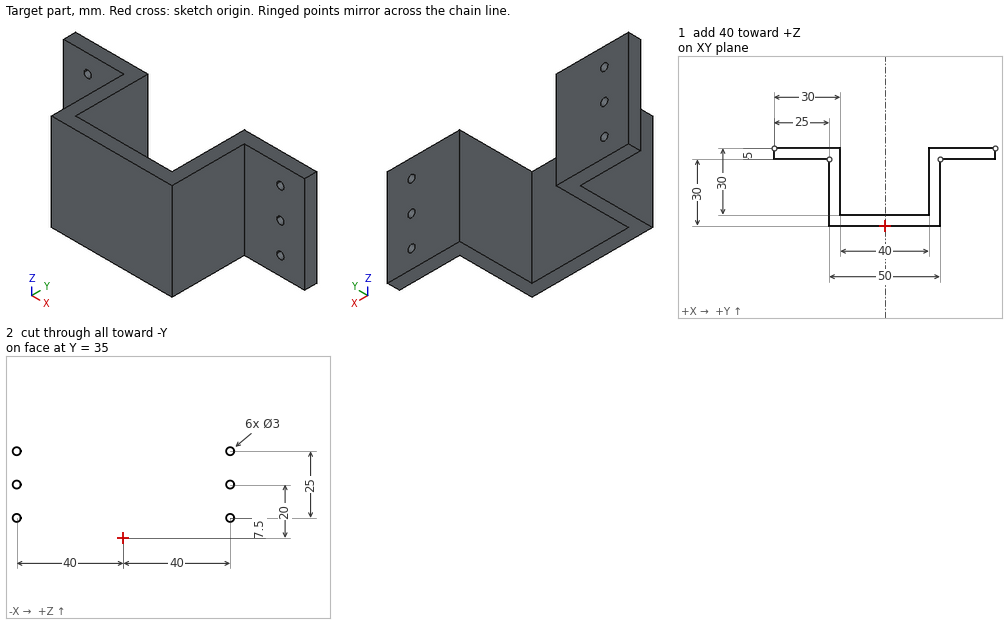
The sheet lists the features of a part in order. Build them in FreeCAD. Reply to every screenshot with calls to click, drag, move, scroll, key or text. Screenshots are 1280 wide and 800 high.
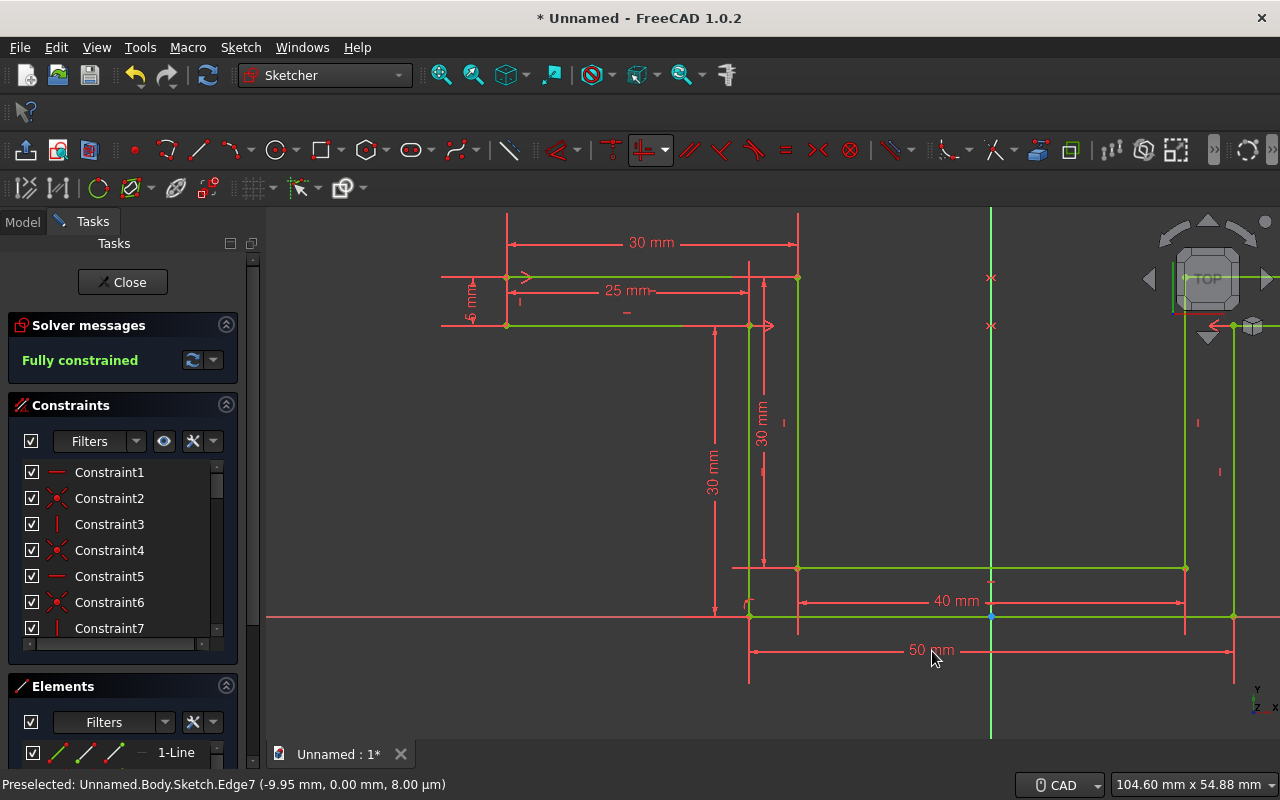
click(123, 282)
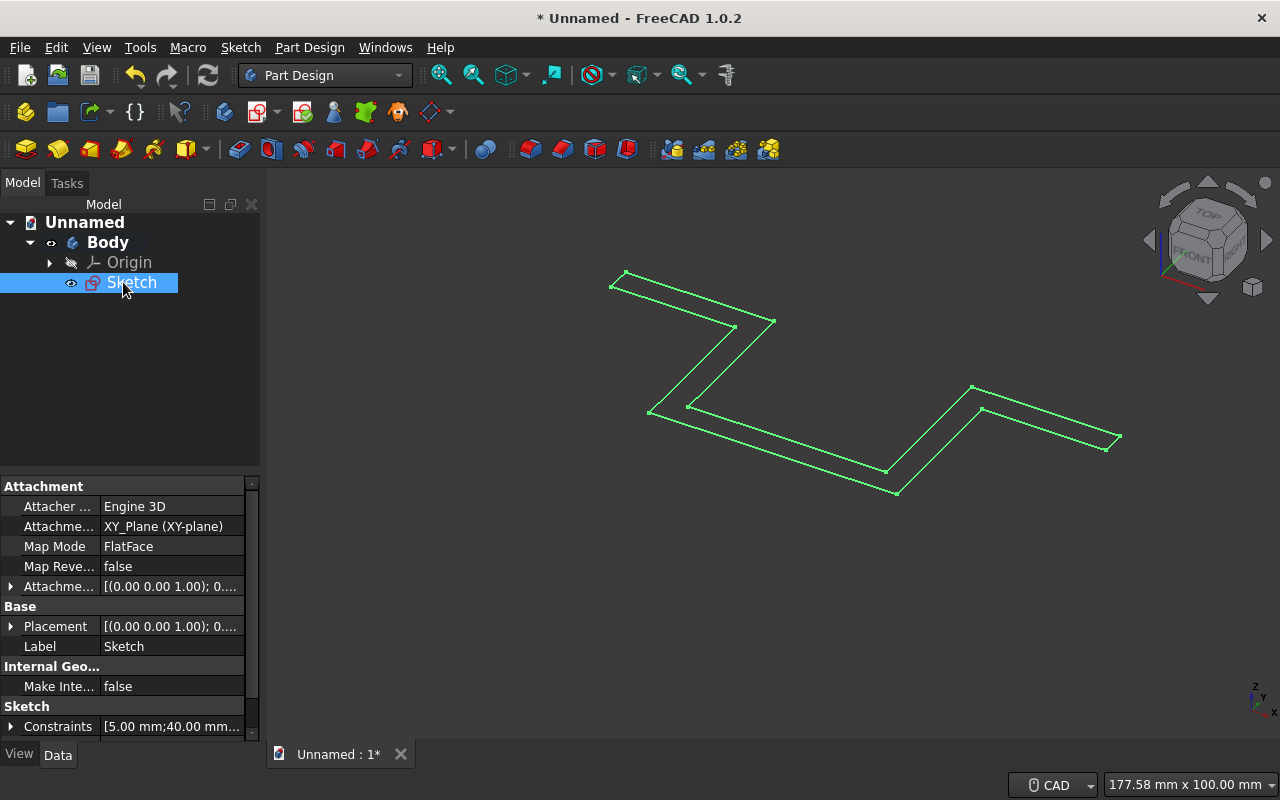
click(26, 150)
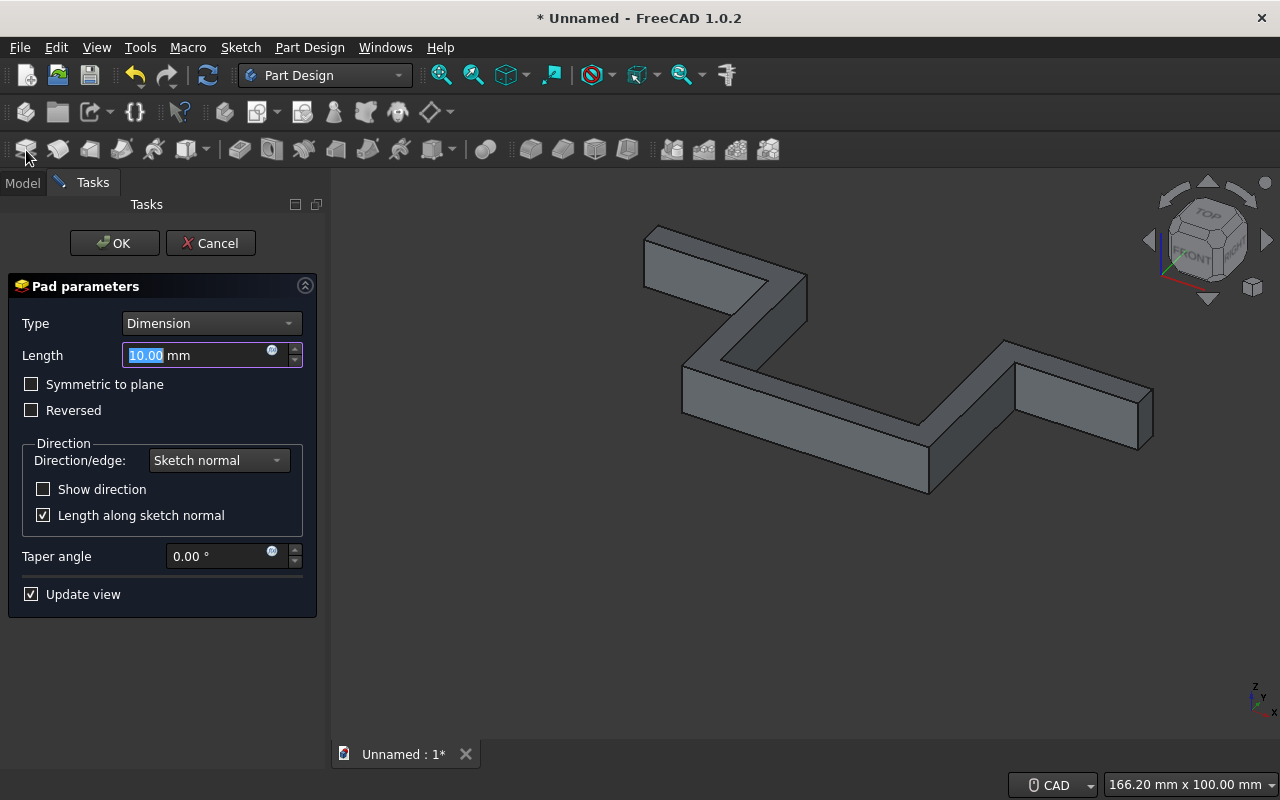
text(40)
key(Tab)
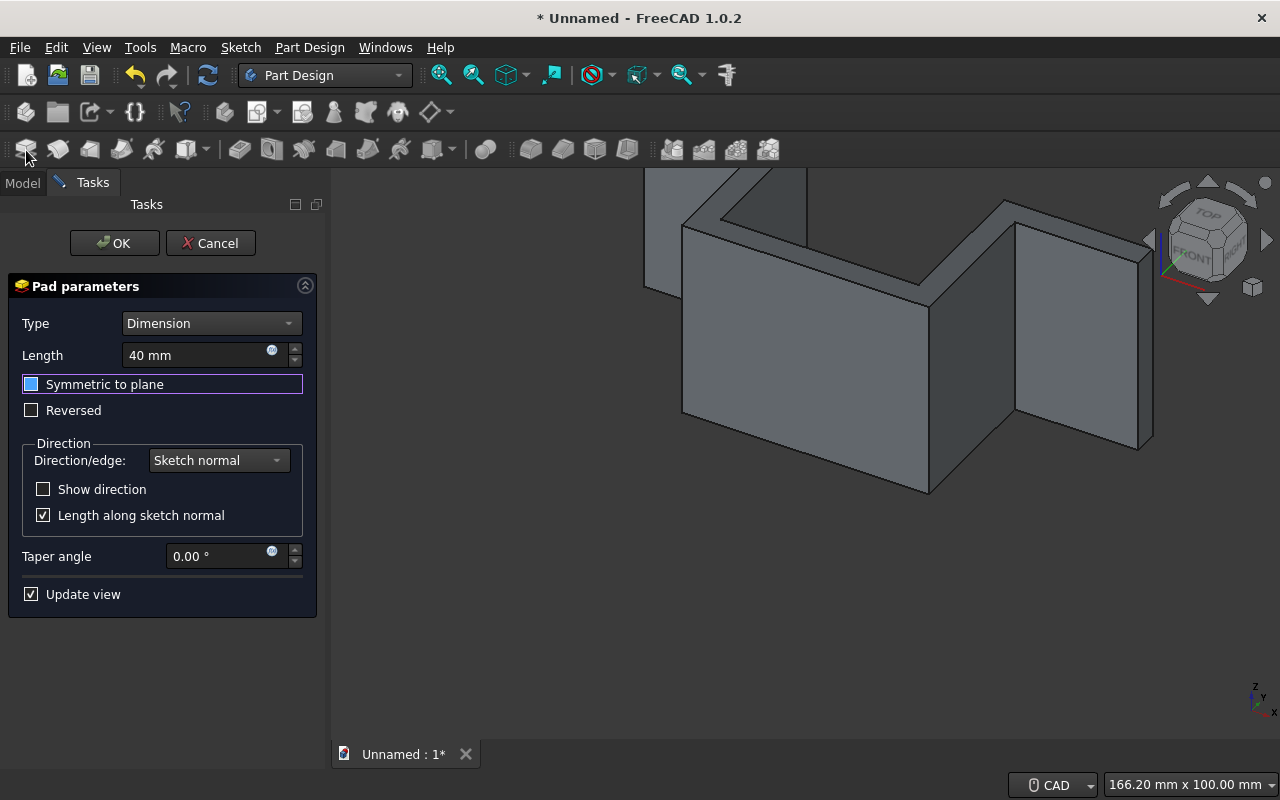
click(115, 243)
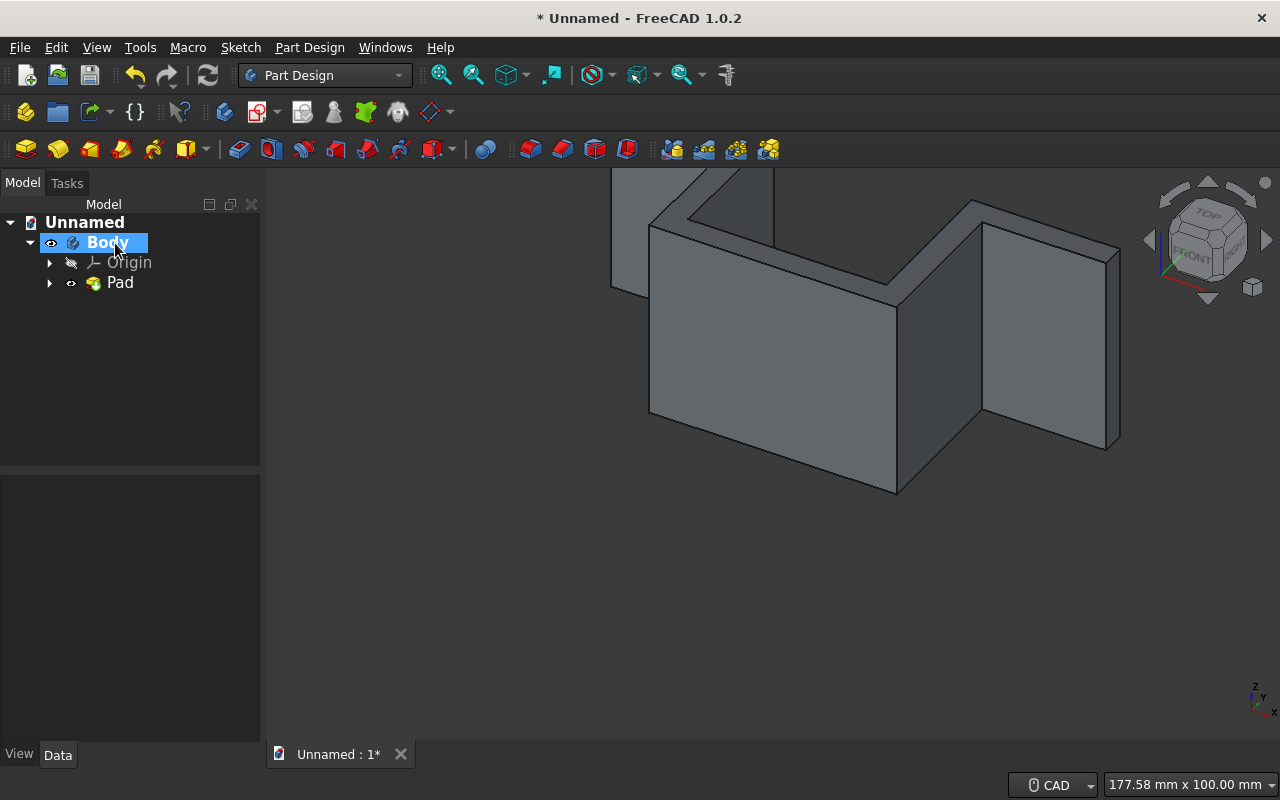
key(v)
key(f)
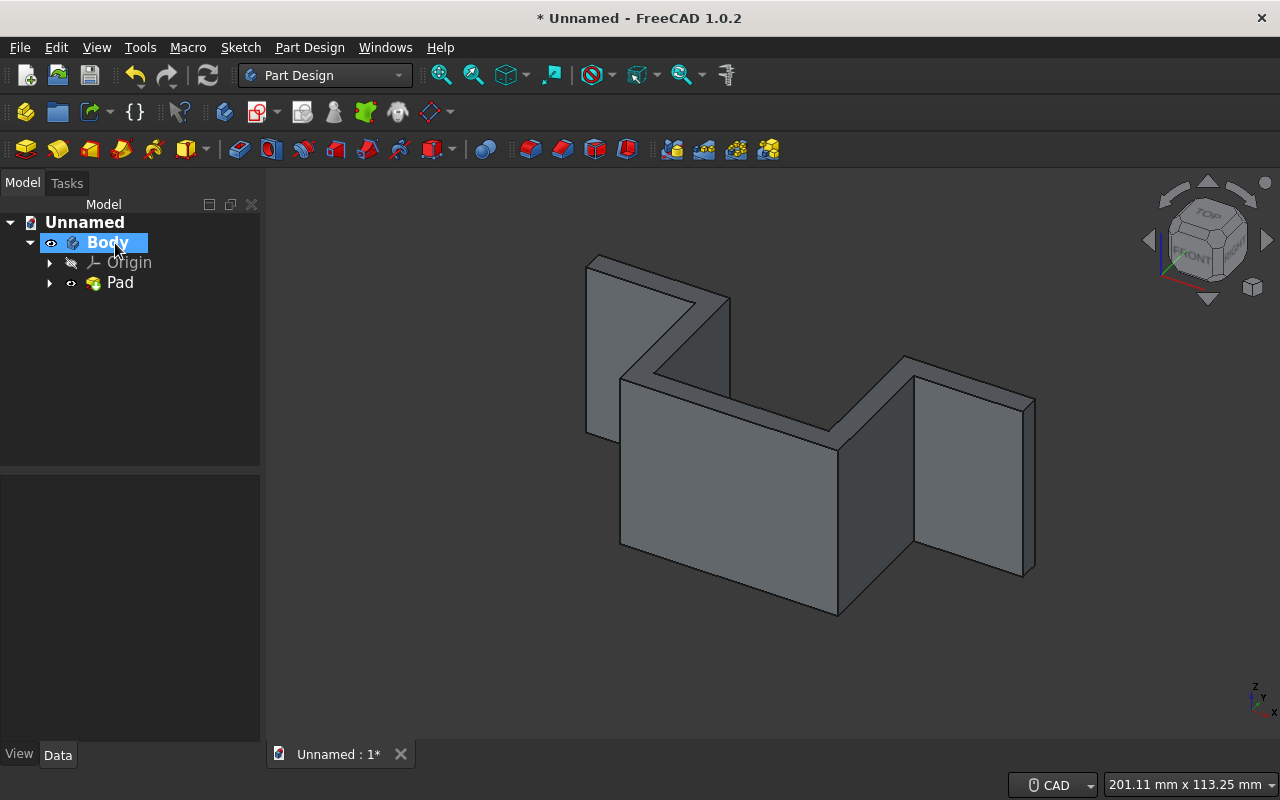
key(4)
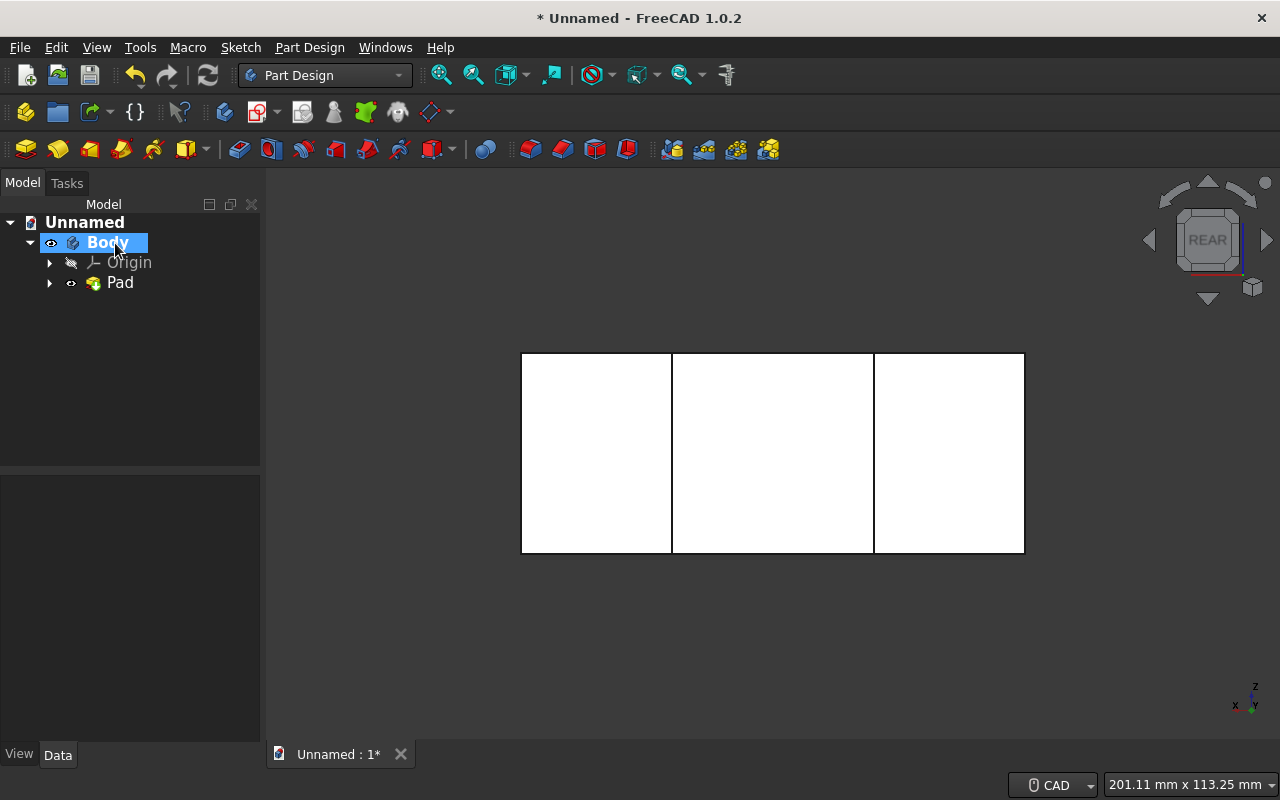
click(949, 453)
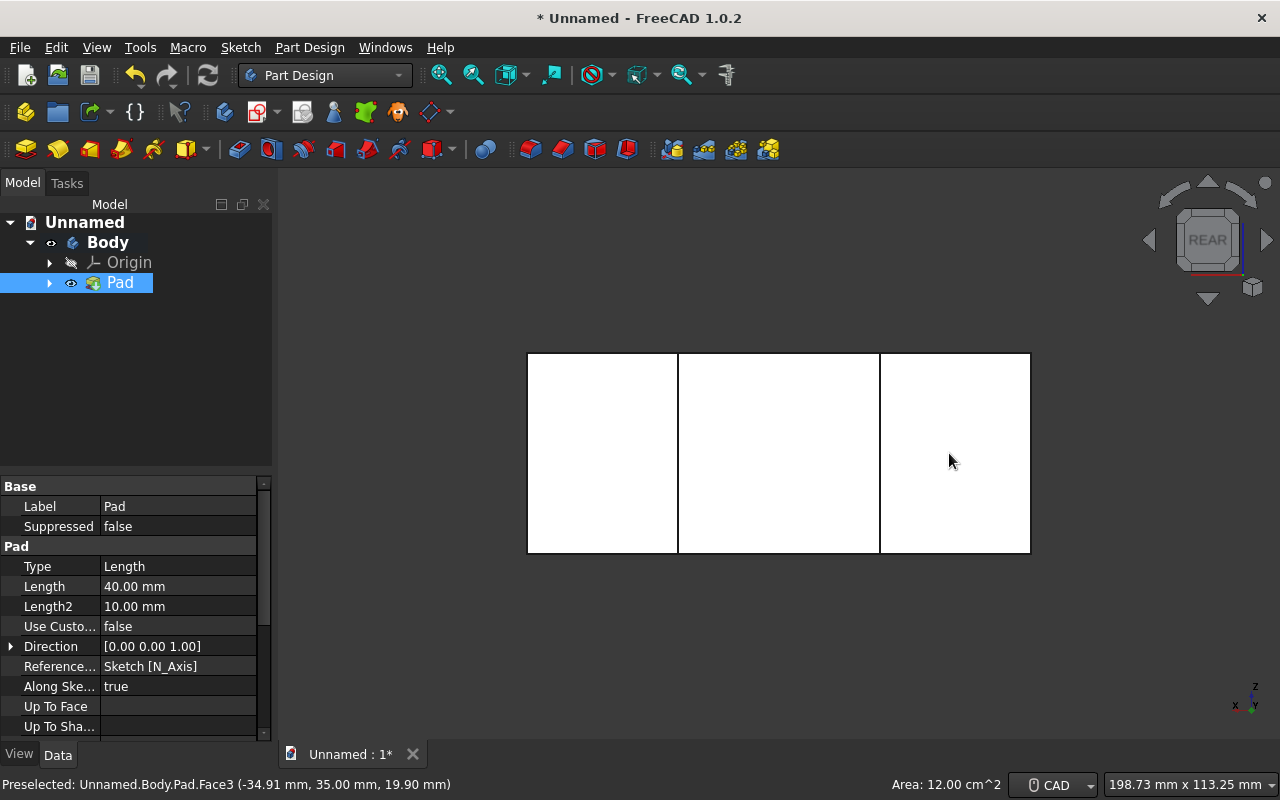
click(258, 112)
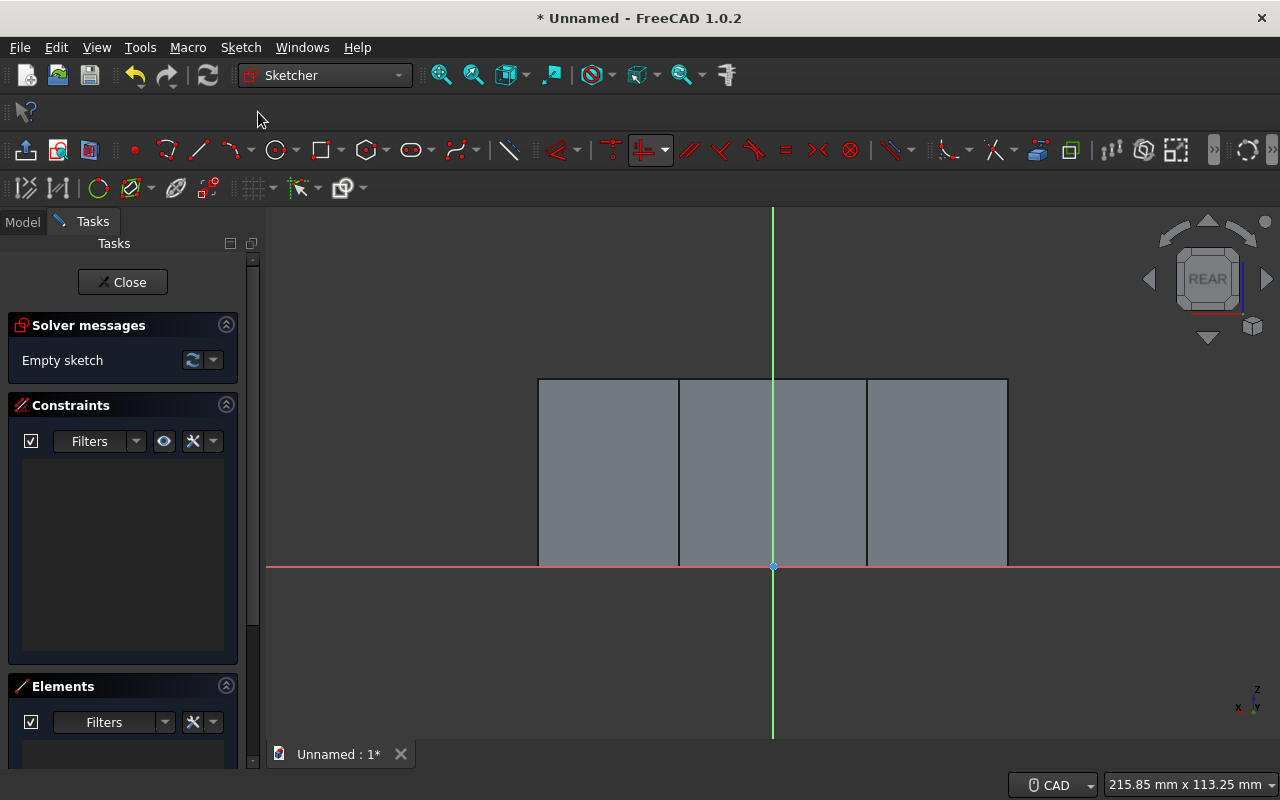
scroll(912, 516, up, 2)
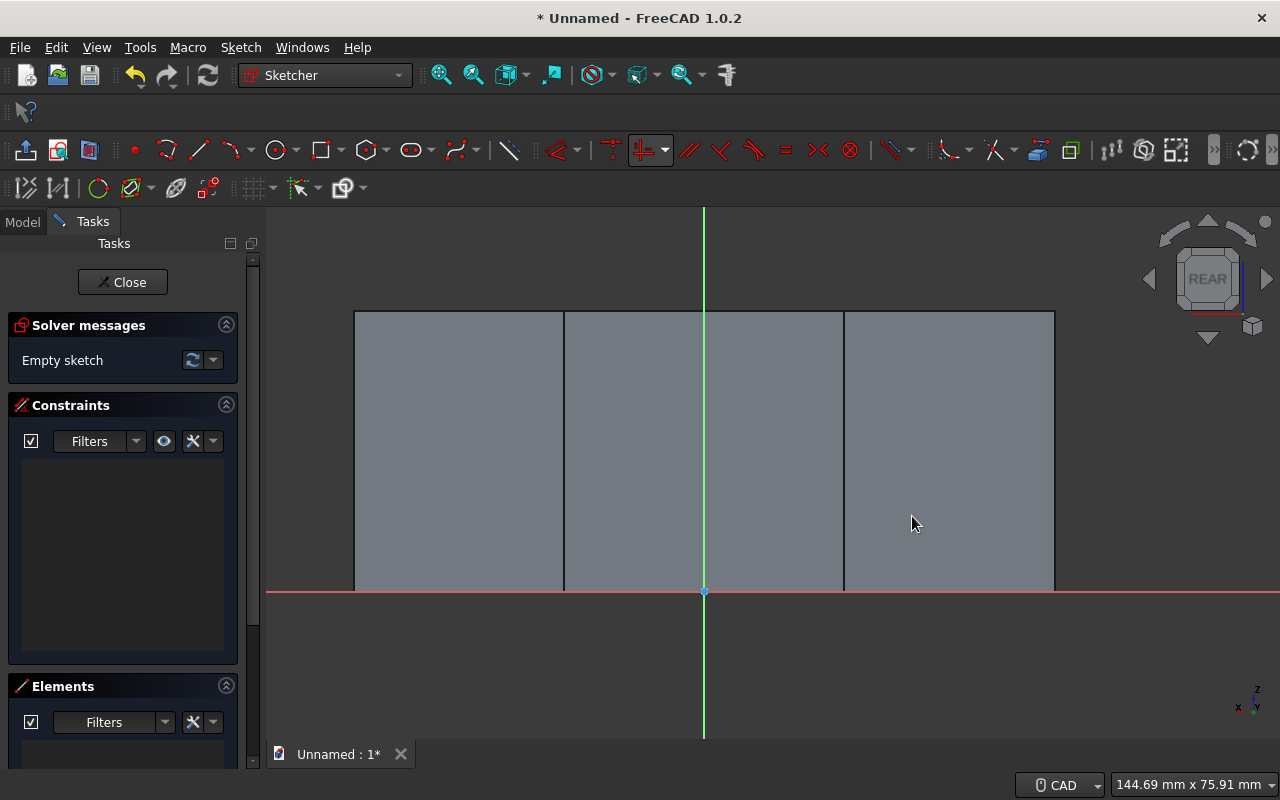
key(g)
key(c)